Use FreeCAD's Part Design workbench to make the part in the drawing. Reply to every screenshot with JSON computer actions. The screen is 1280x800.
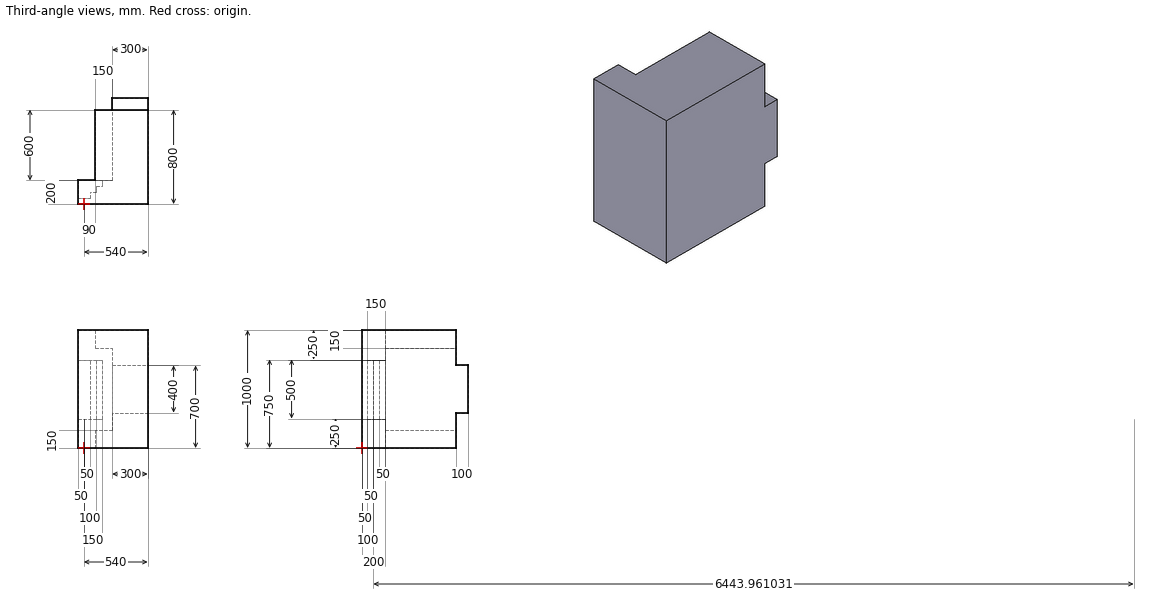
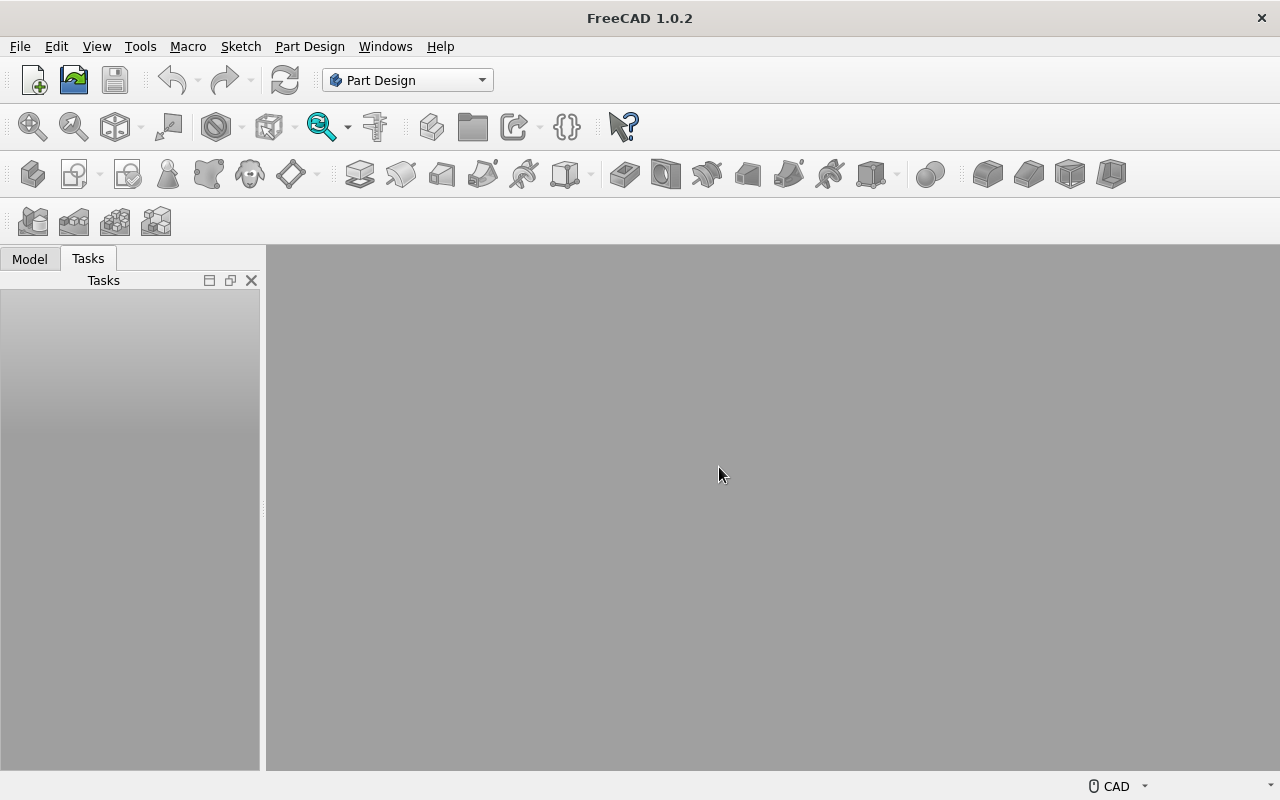
{"action": "left_click", "coordinate": [33, 80]}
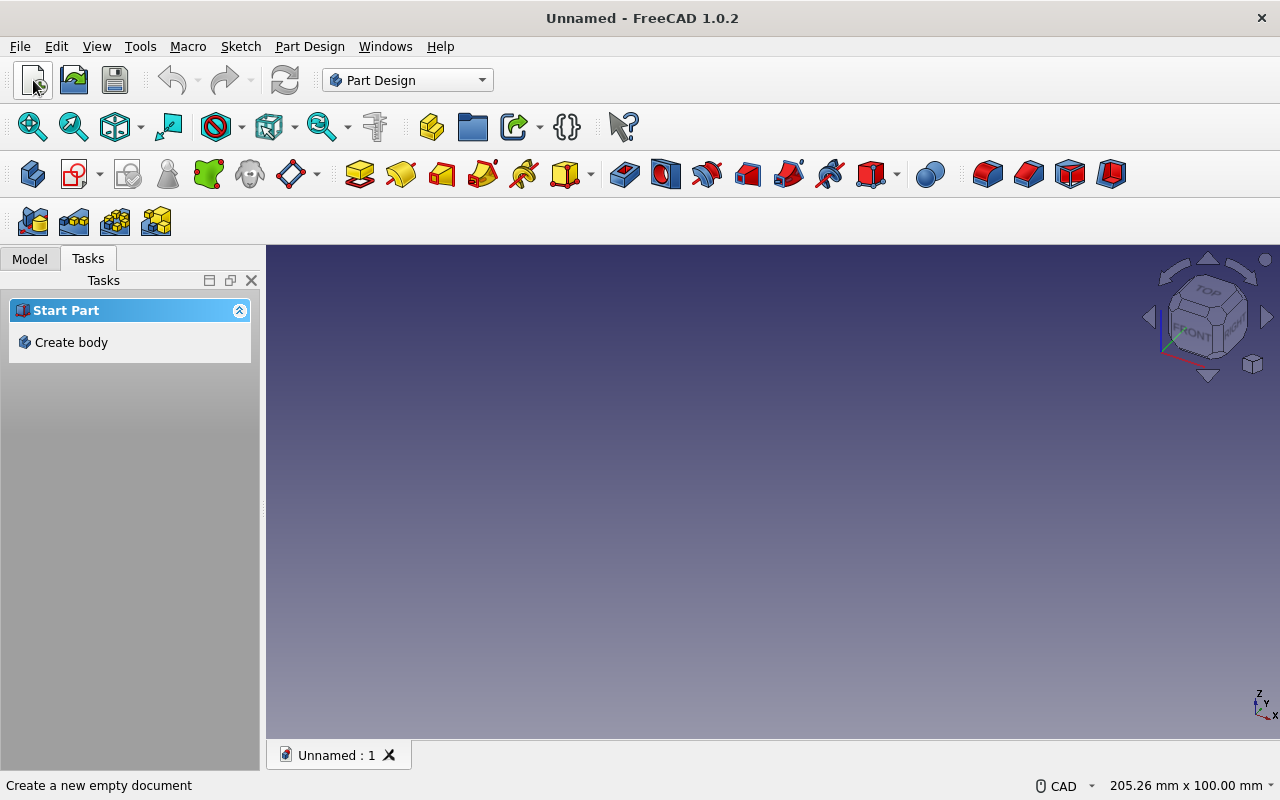
{"action": "left_click", "coordinate": [74, 174]}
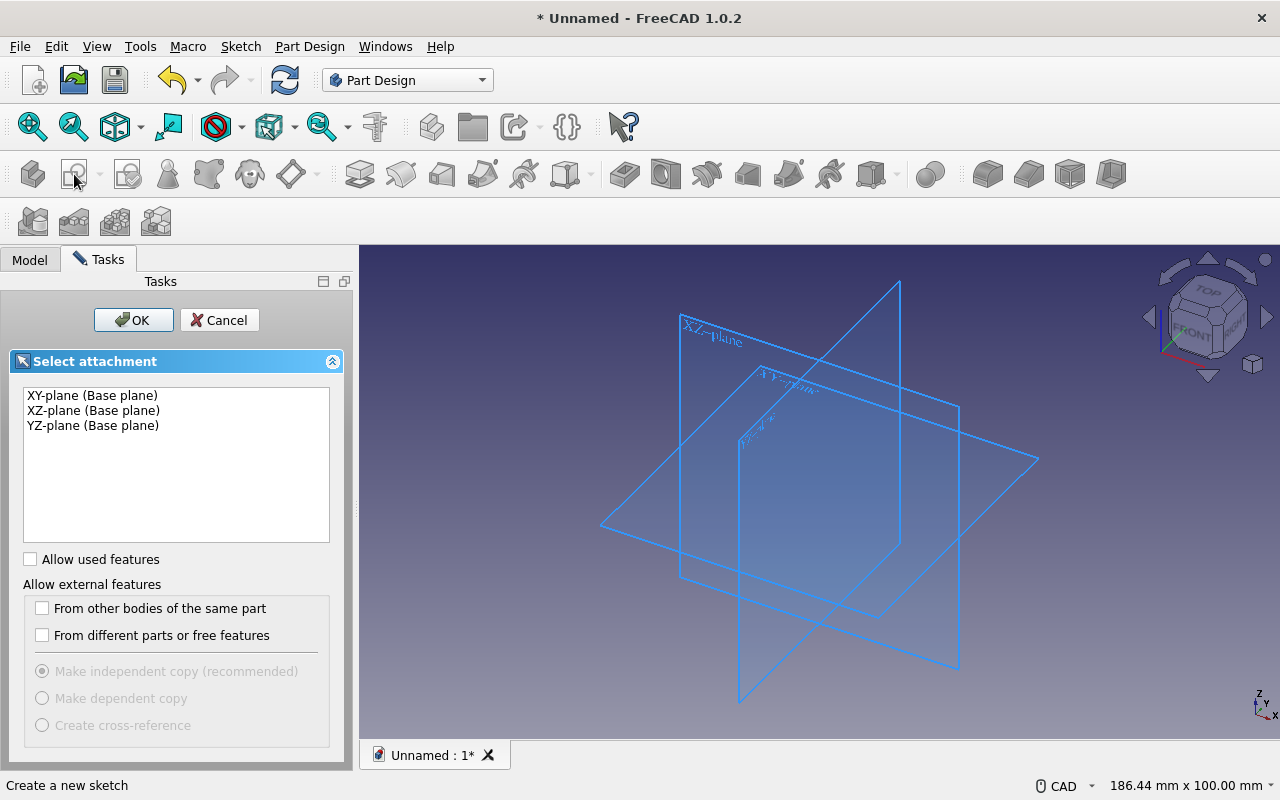
{"action": "left_click", "coordinate": [84, 396]}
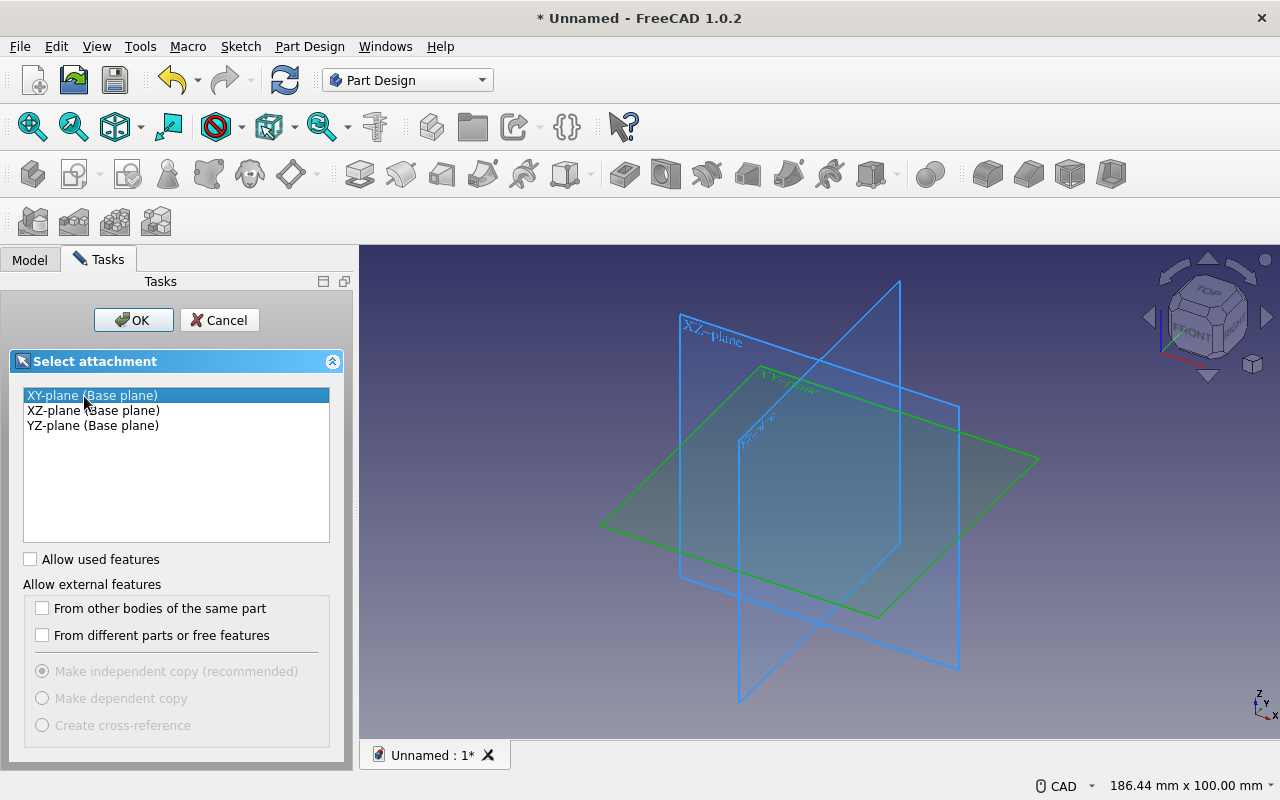
{"action": "left_click", "coordinate": [134, 320]}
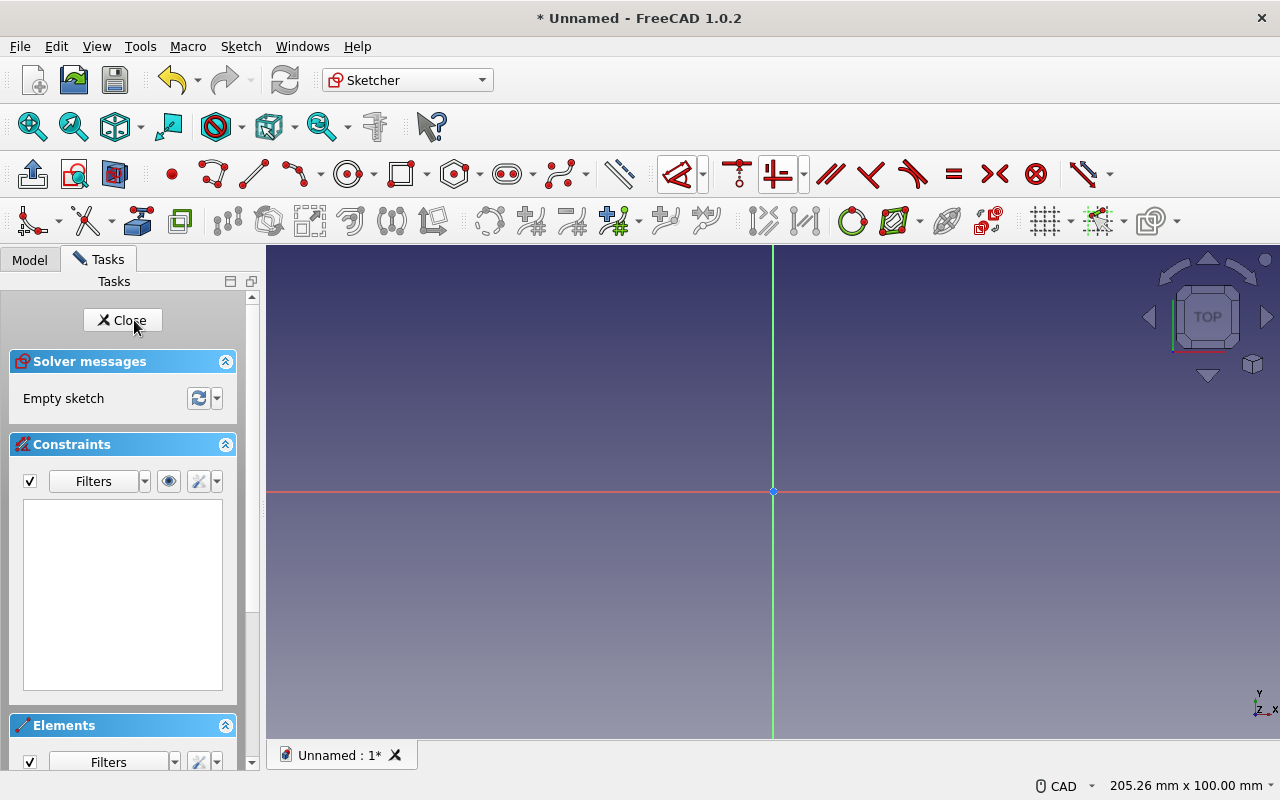
{"action": "scroll", "coordinate": [592, 651], "scroll_direction": "down", "scroll_amount": 13}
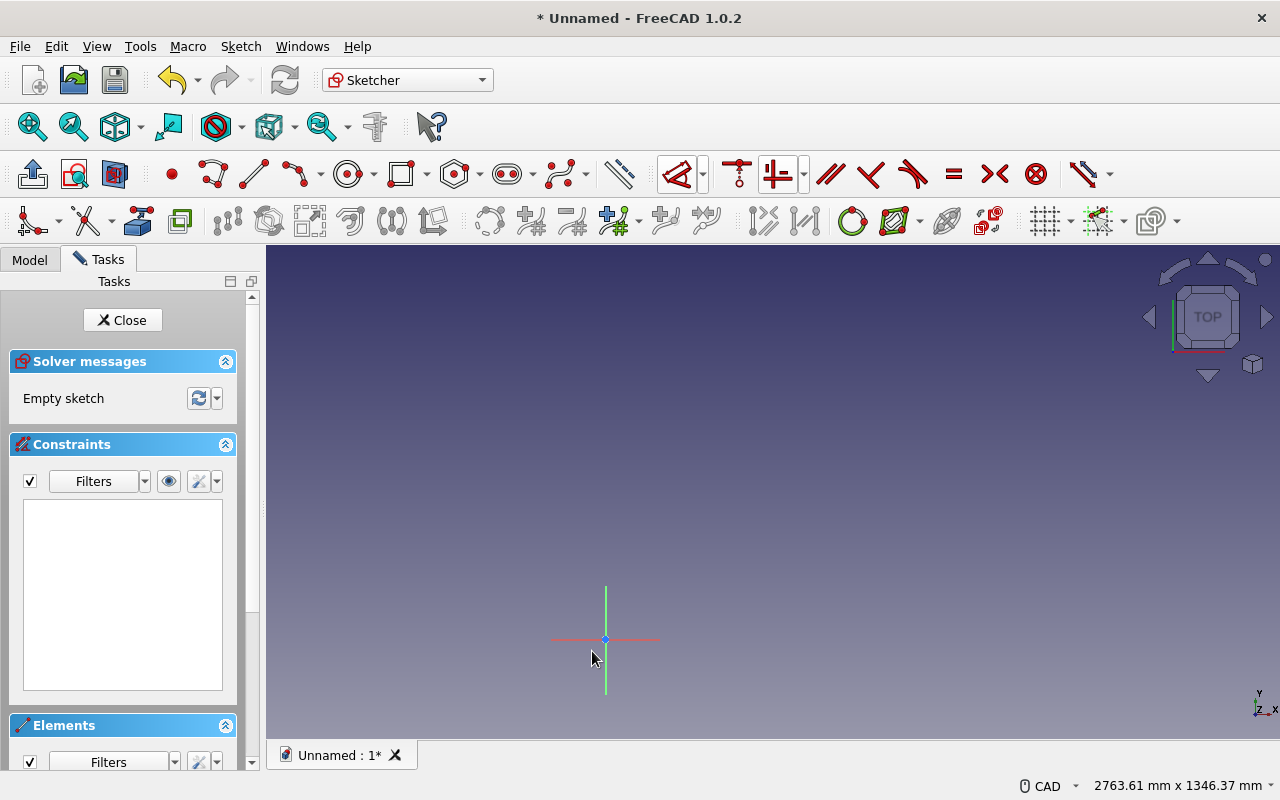
{"action": "left_click", "coordinate": [213, 174]}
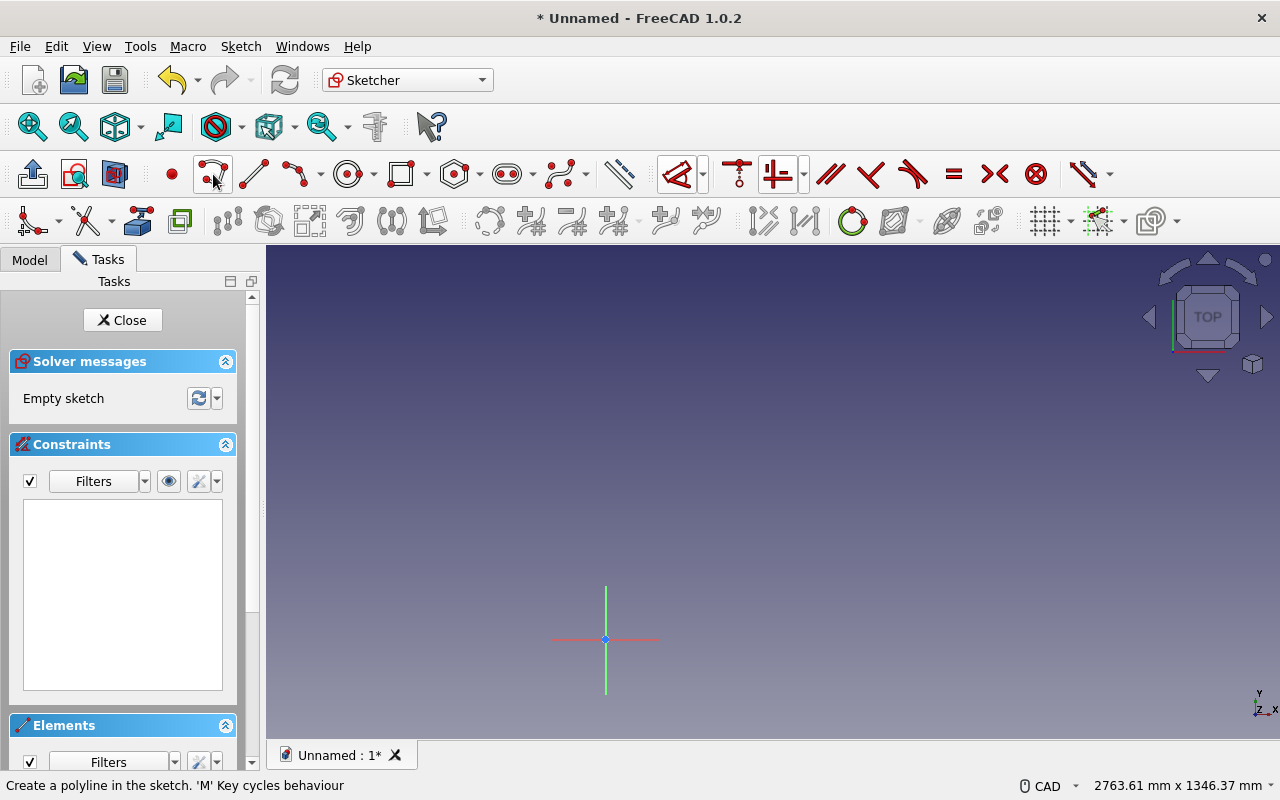
{"action": "left_click", "coordinate": [606, 640]}
{"action": "left_click", "coordinate": [804, 631]}
{"action": "left_click", "coordinate": [804, 346]}
{"action": "left_click", "coordinate": [694, 346]}
{"action": "left_click", "coordinate": [694, 567]}
{"action": "left_click", "coordinate": [615, 567]}
{"action": "left_click", "coordinate": [606, 640]}
{"action": "key", "text": "Escape"}
{"action": "key", "text": "Escape"}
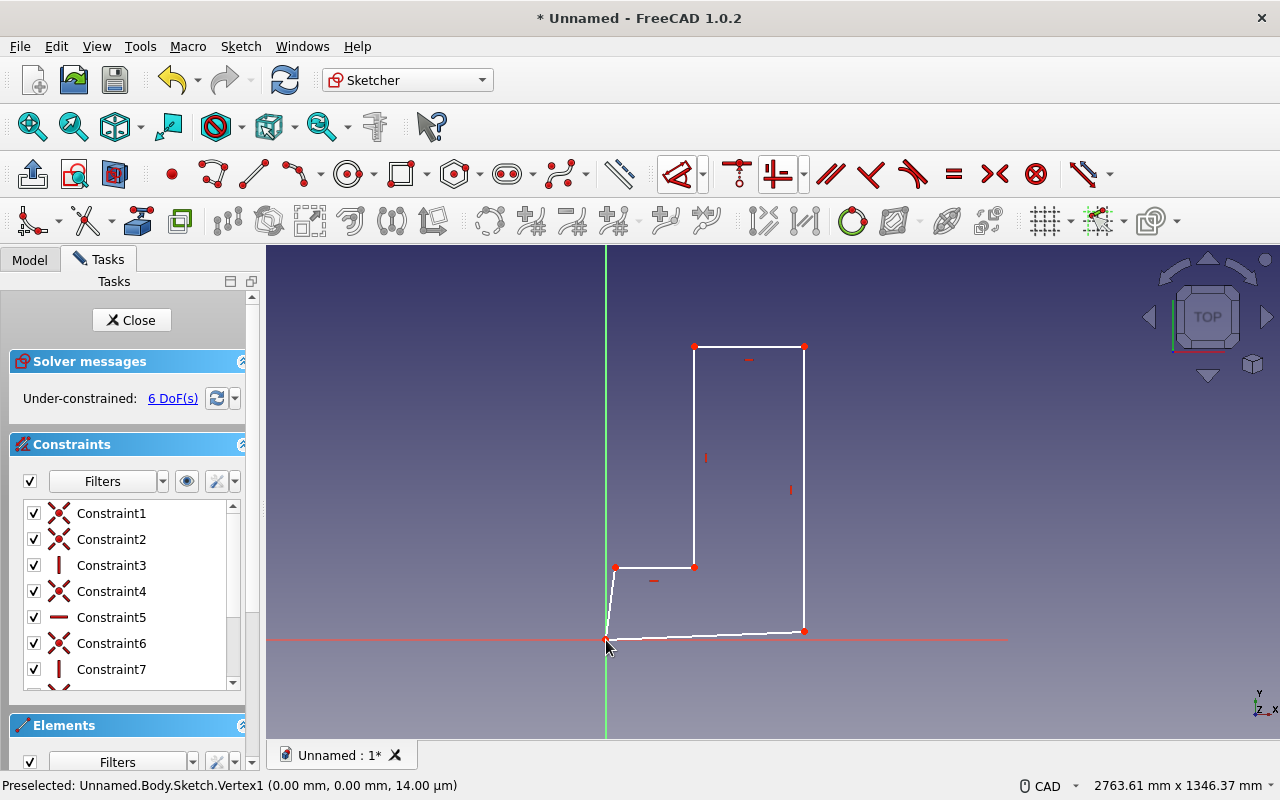
{"action": "left_click", "coordinate": [665, 638]}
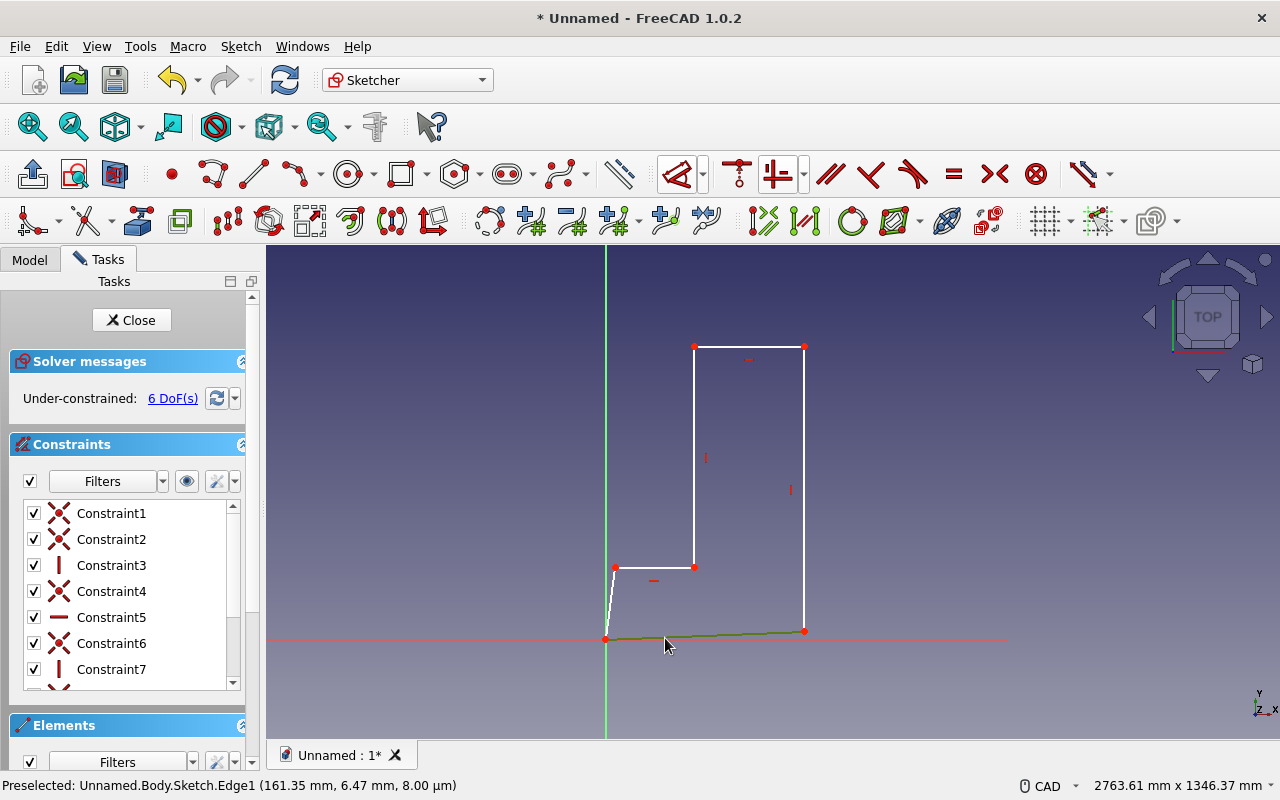
{"action": "left_click", "coordinate": [804, 174]}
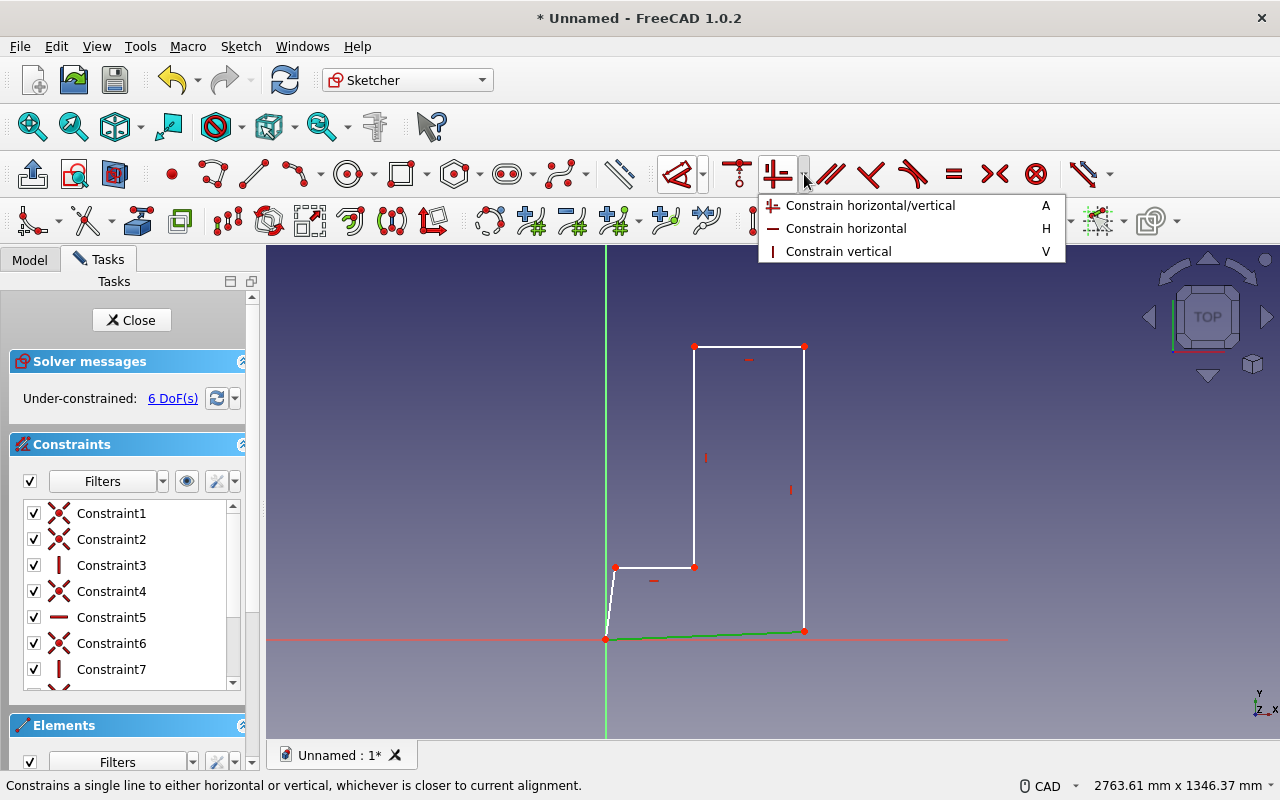
{"action": "left_click", "coordinate": [912, 228]}